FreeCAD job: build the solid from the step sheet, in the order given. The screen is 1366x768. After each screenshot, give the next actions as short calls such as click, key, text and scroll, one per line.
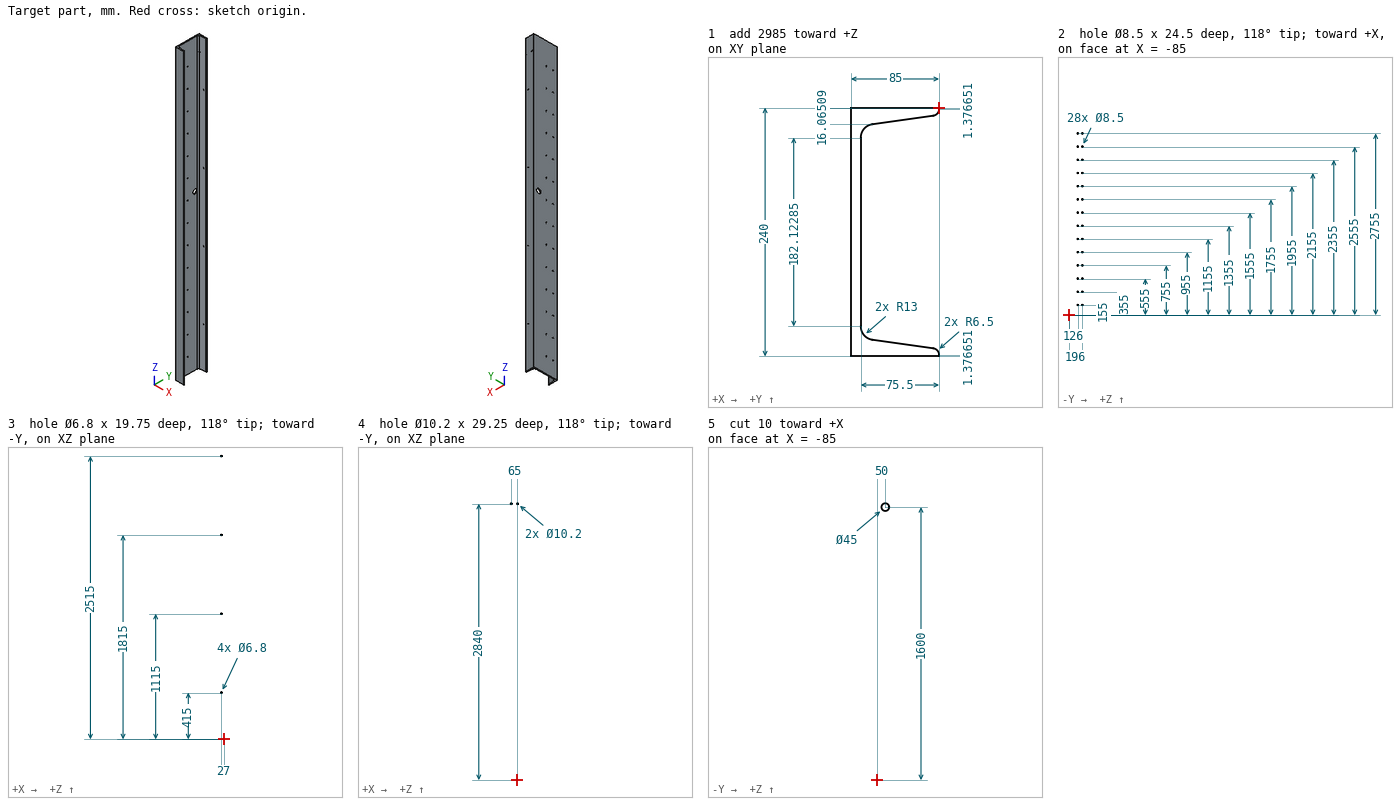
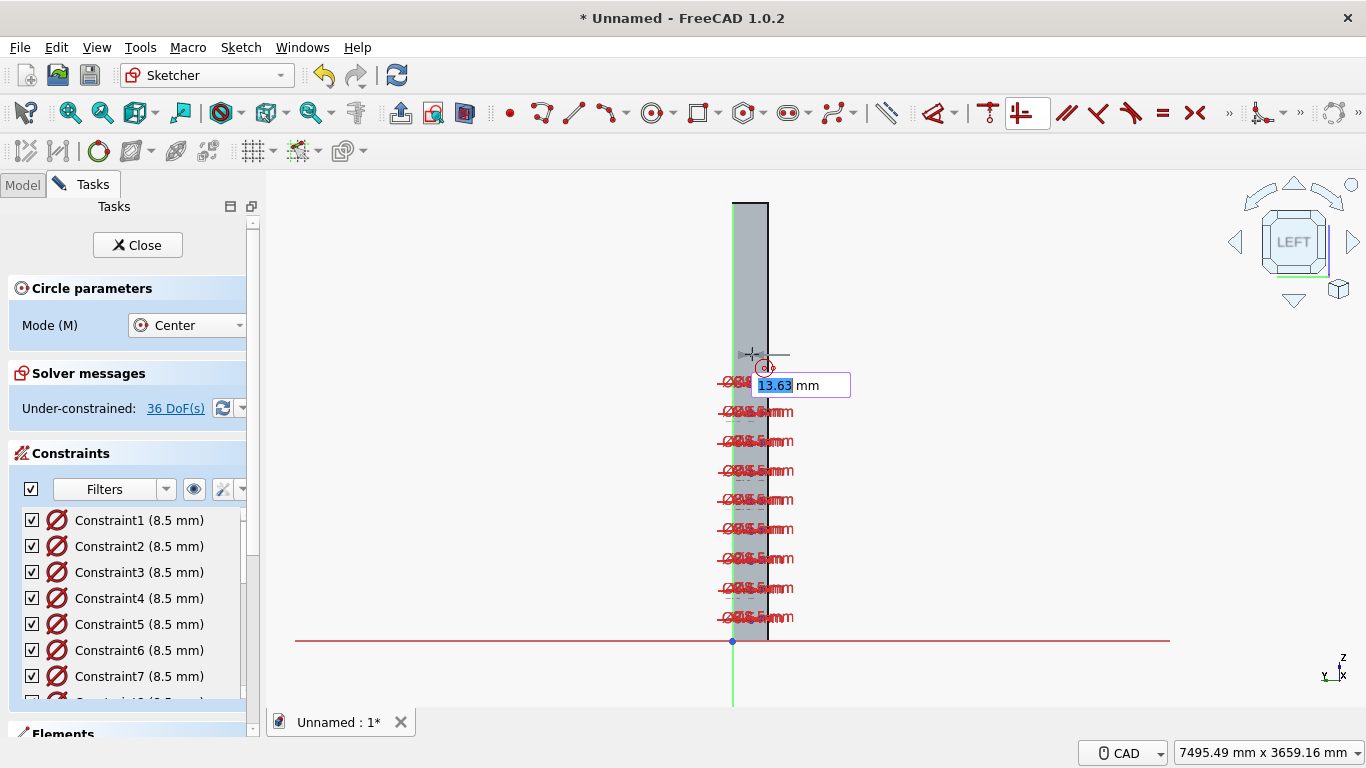
text(8.5)
key(Return)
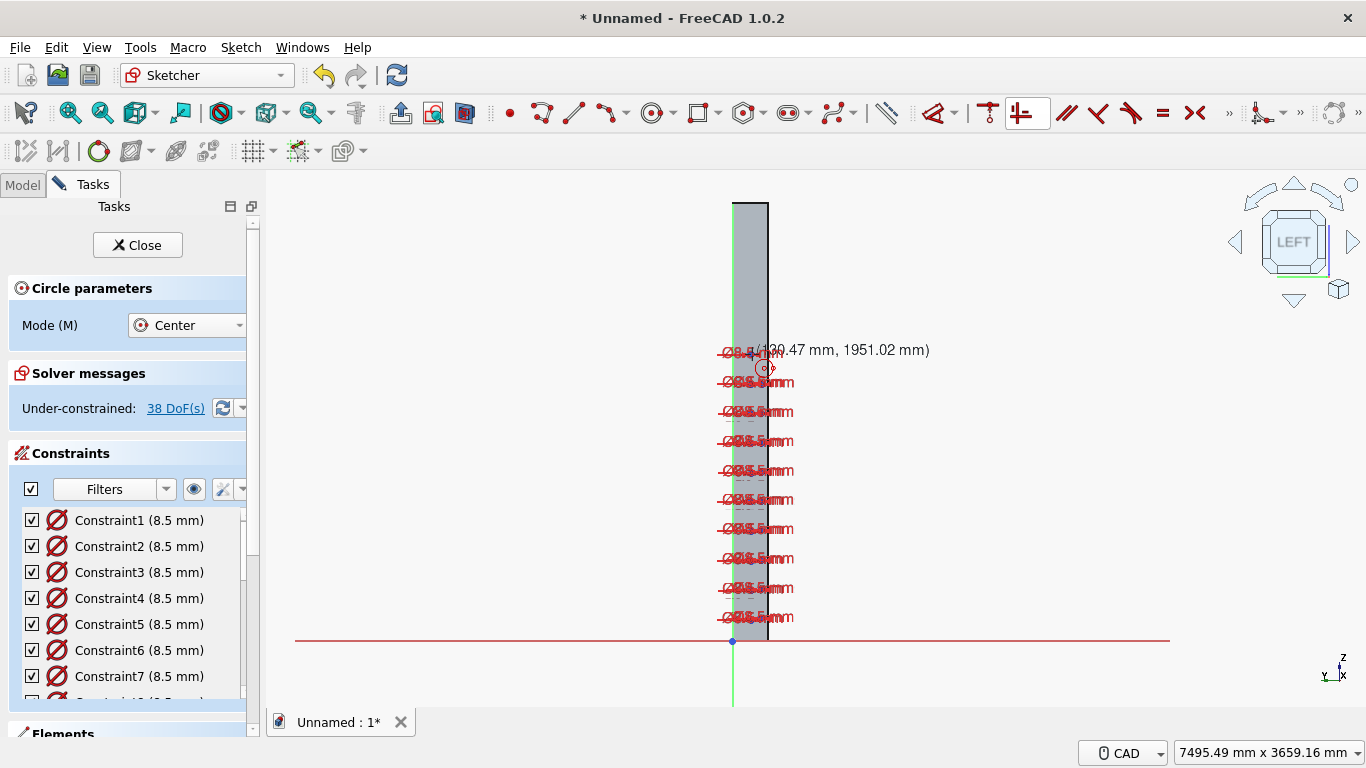
scroll(762, 354, up, 18)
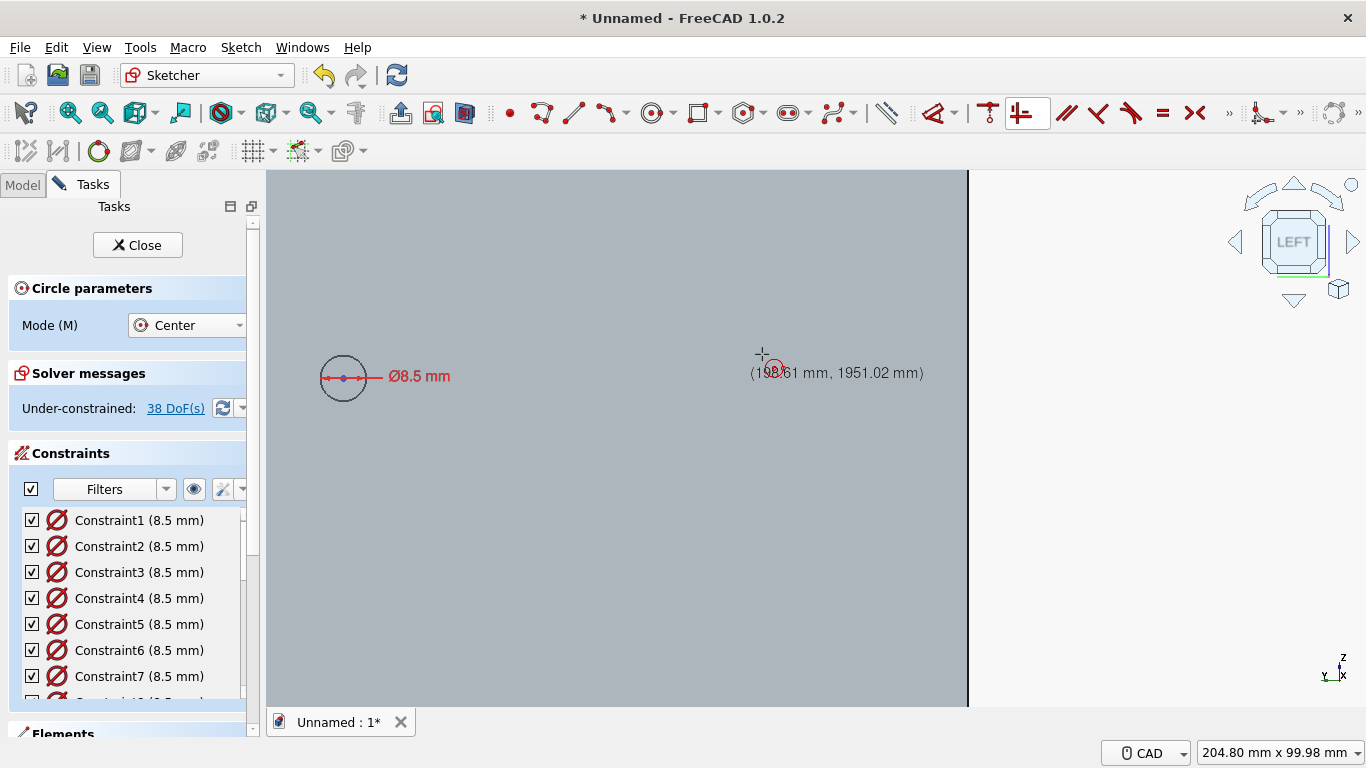
scroll(762, 354, down, 18)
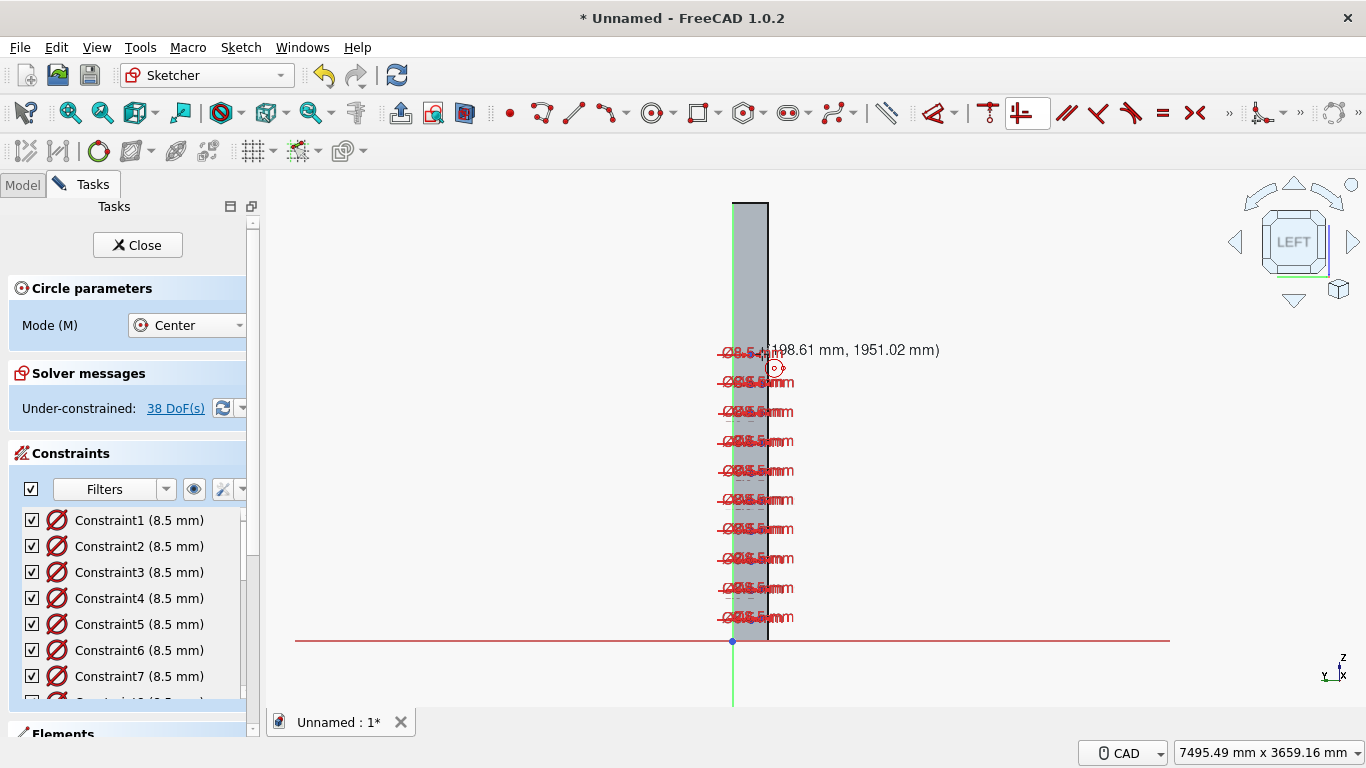
scroll(762, 354, up, 3)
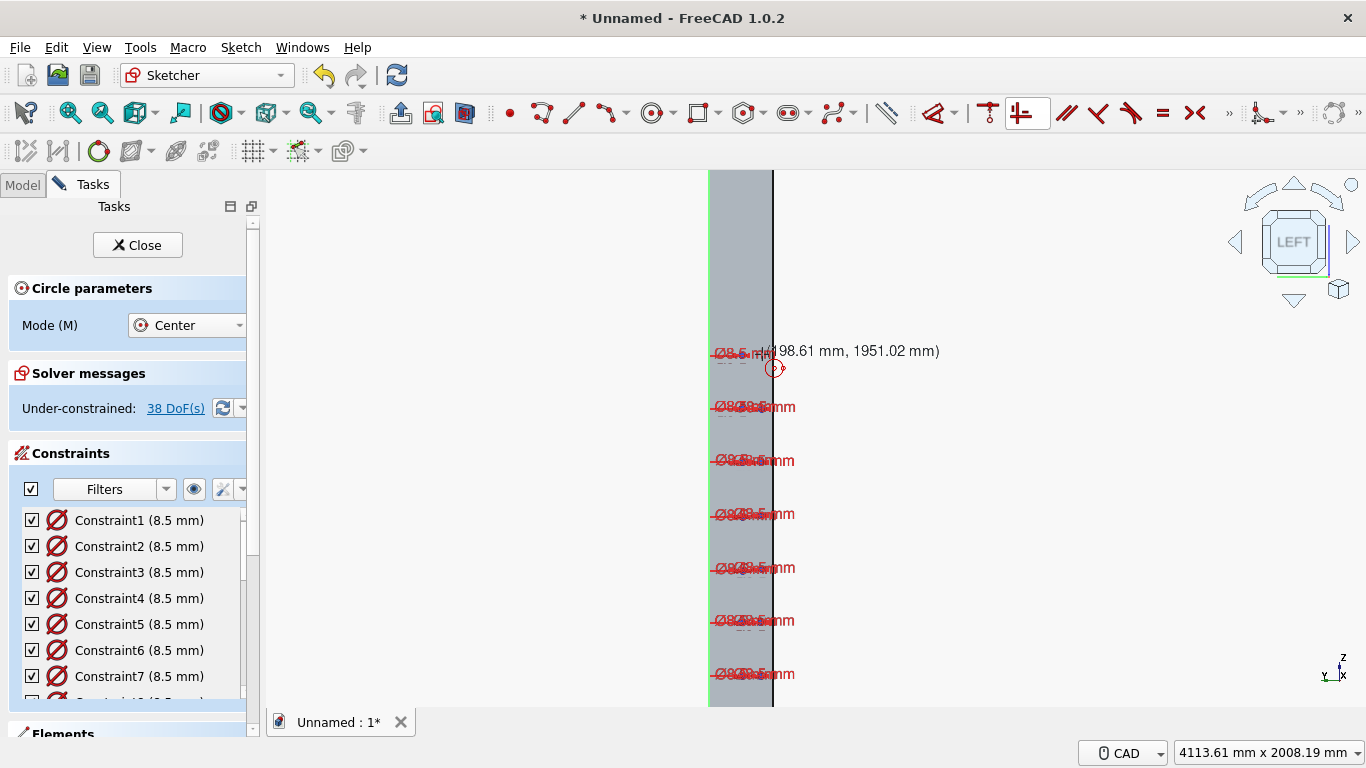
click(761, 354)
move(762, 354)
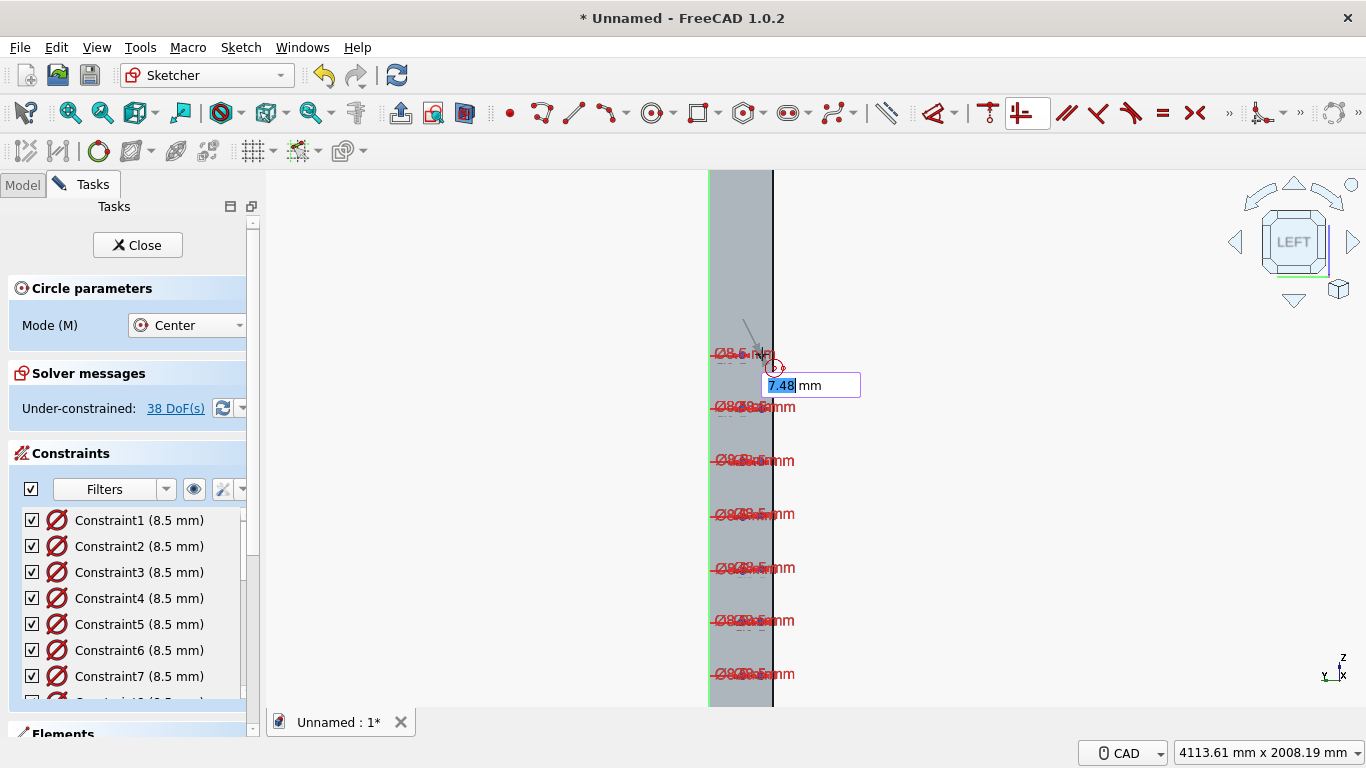
text(8.5)
key(Return)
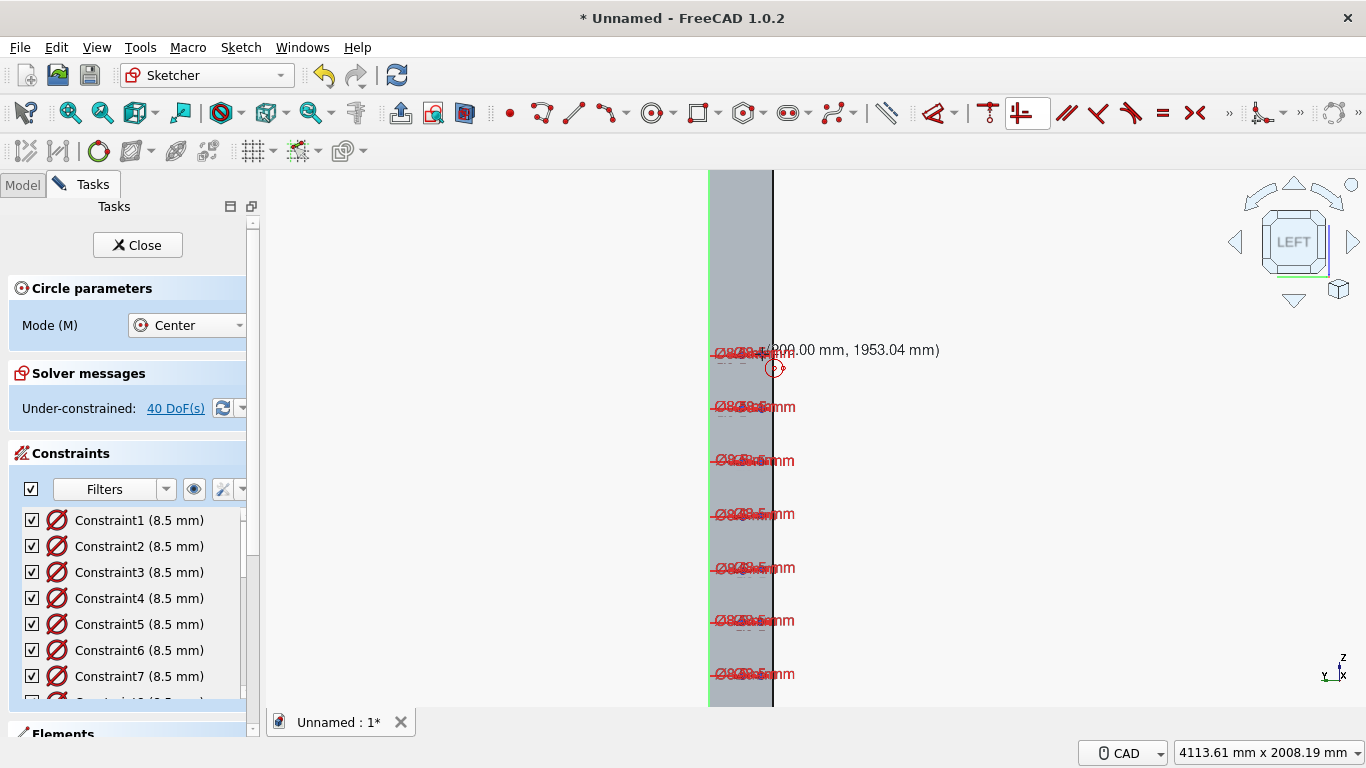
scroll(761, 301, up, 15)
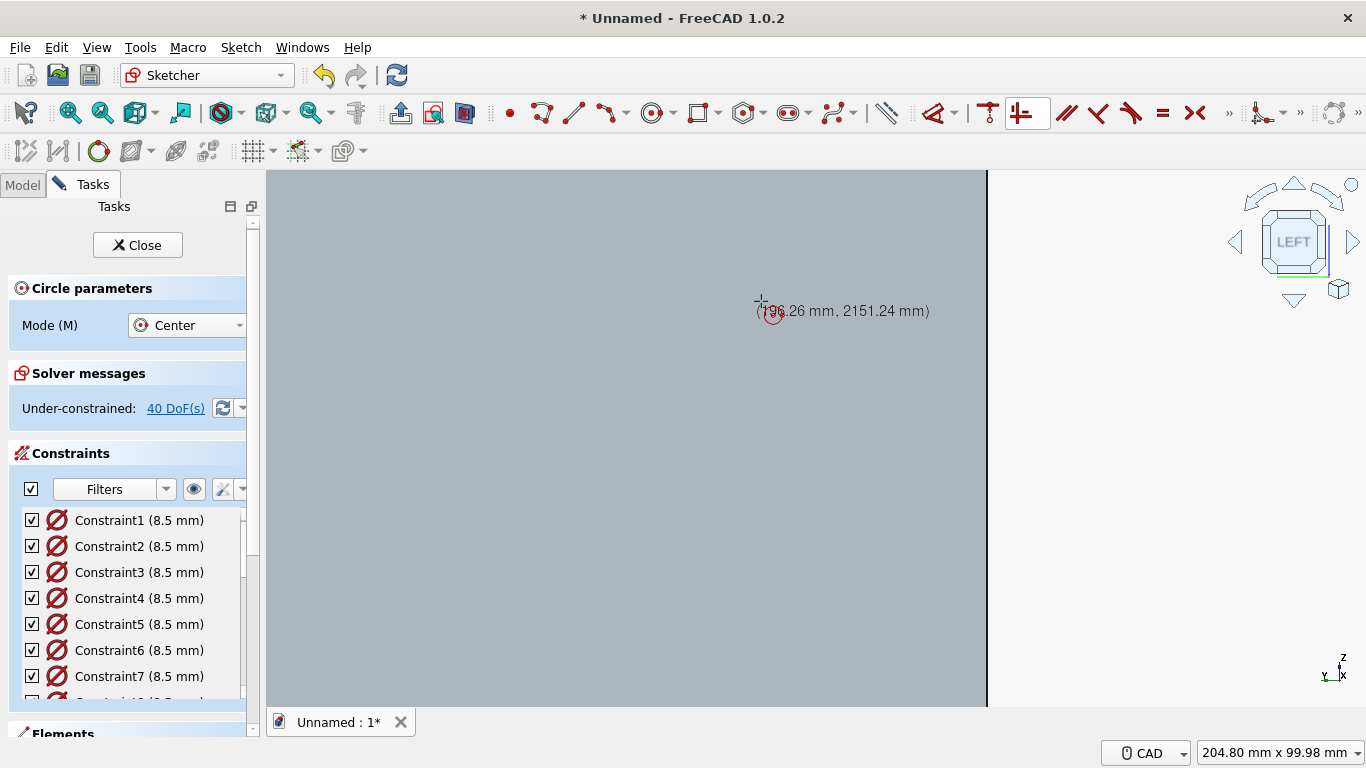
scroll(762, 326, down, 18)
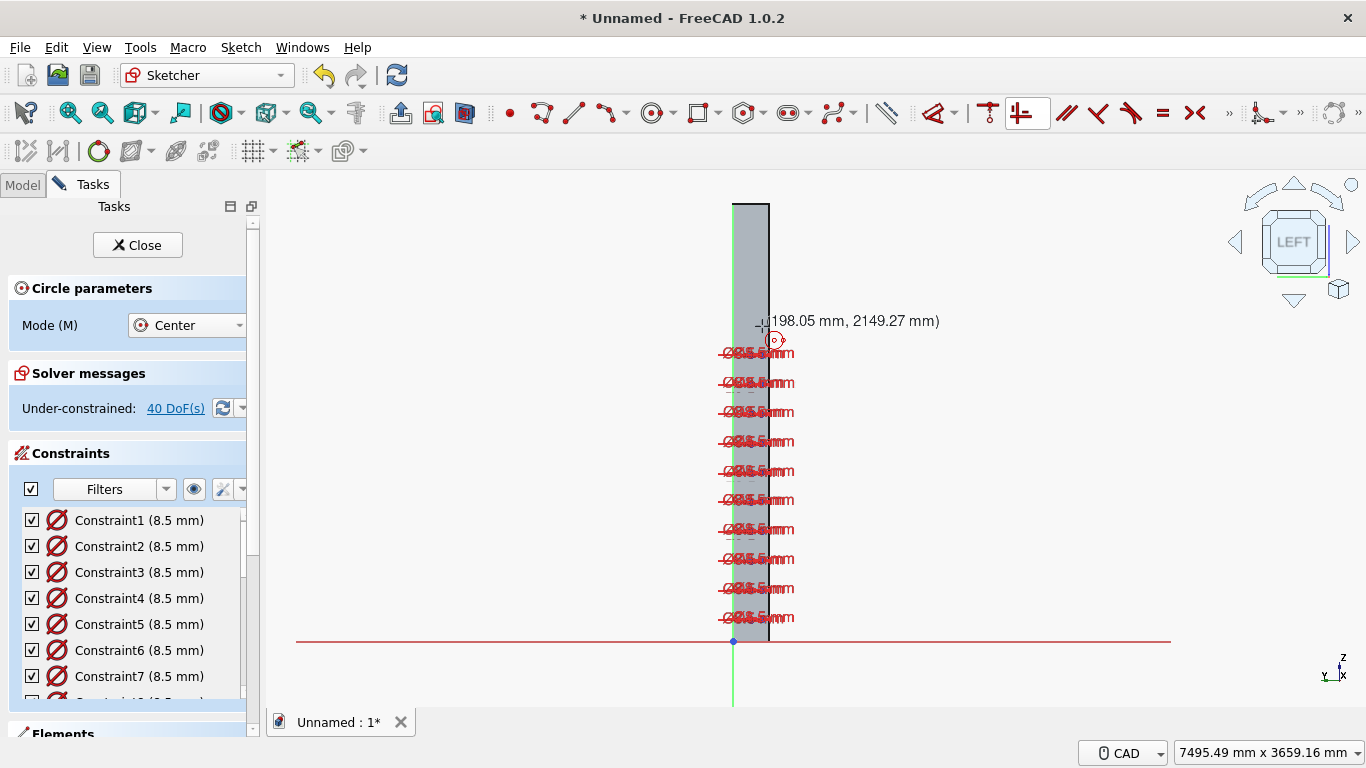
click(762, 325)
move(763, 325)